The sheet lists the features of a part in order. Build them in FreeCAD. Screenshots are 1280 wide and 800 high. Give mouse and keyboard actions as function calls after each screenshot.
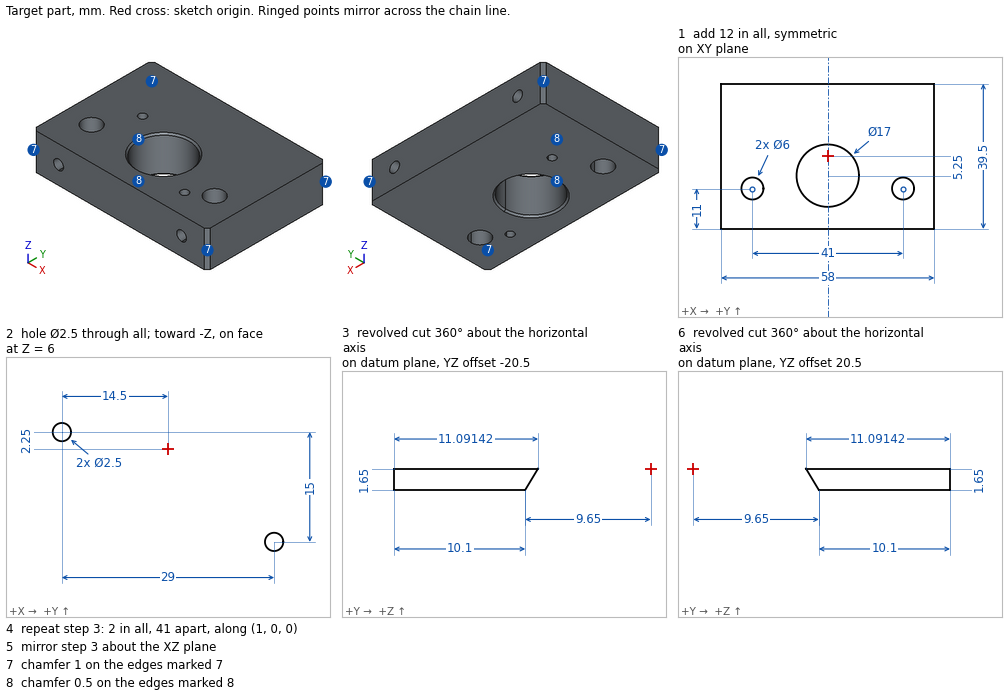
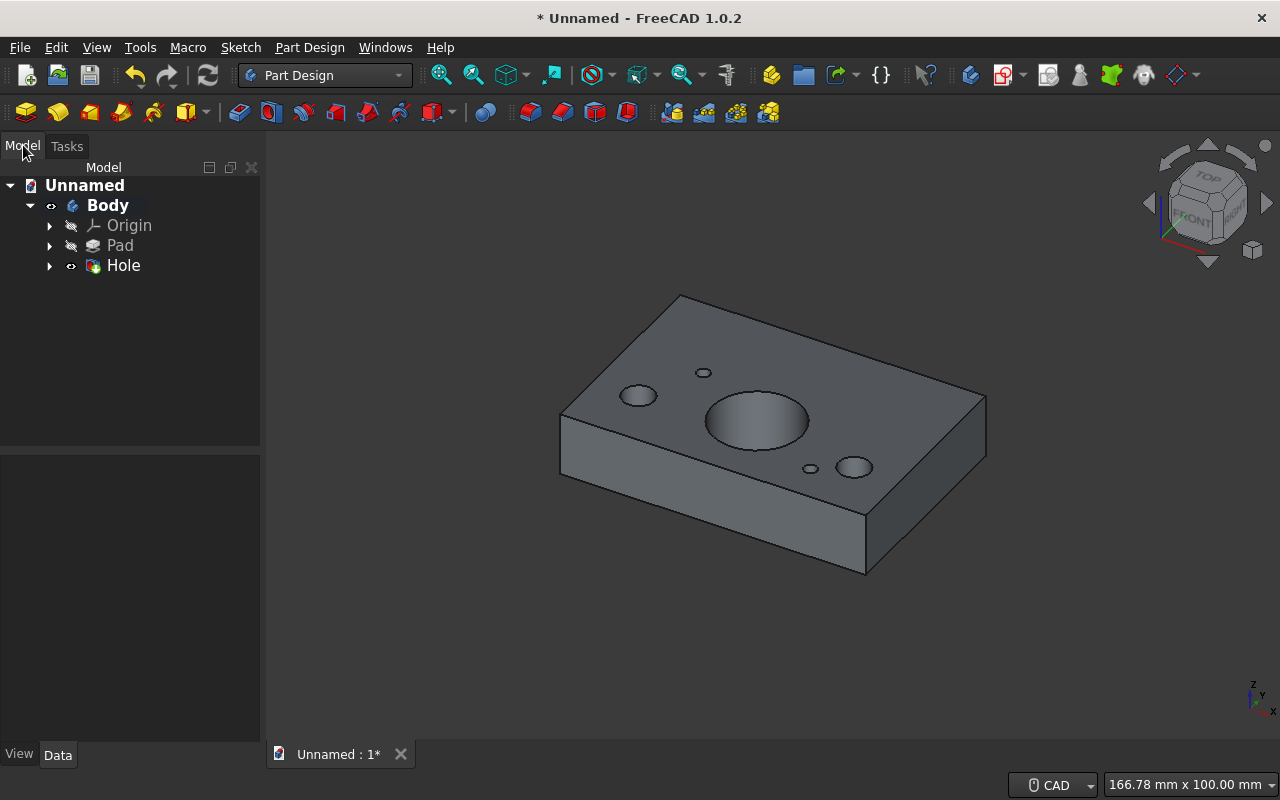
click(50, 226)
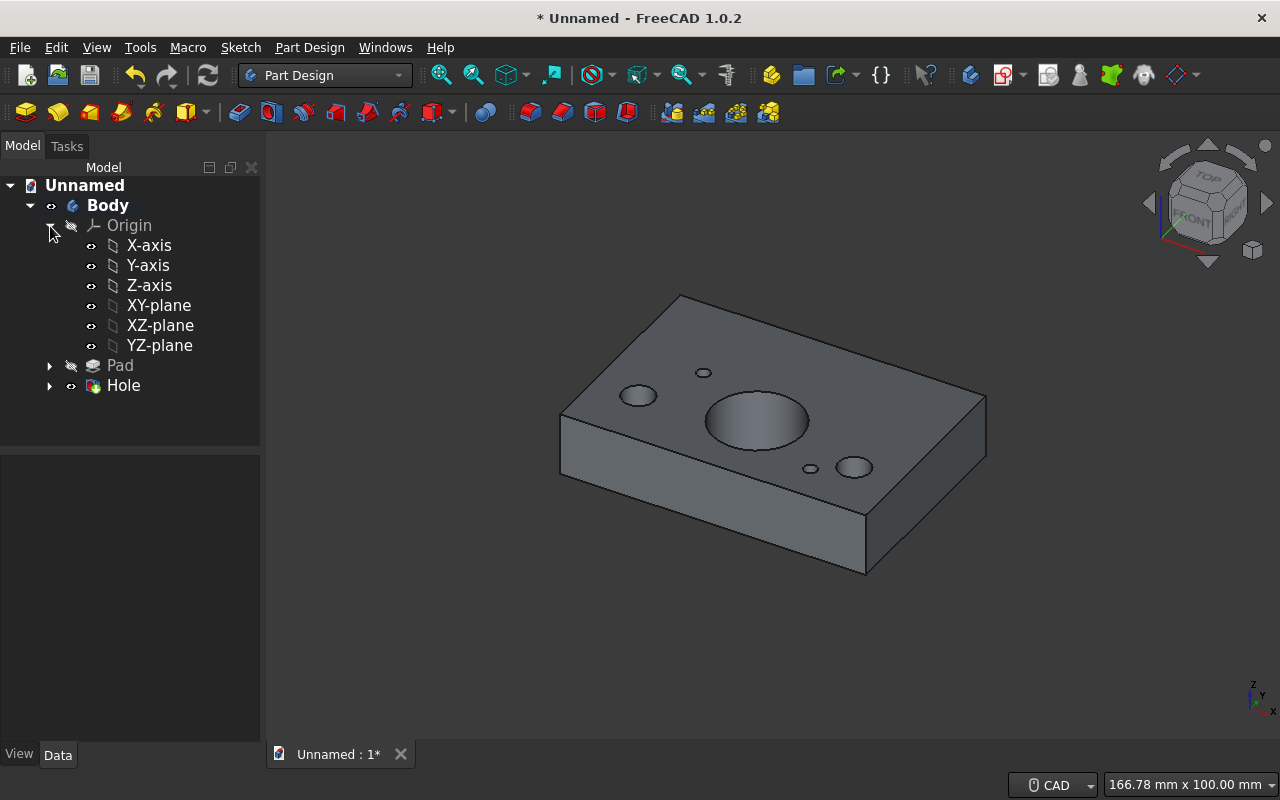
click(136, 346)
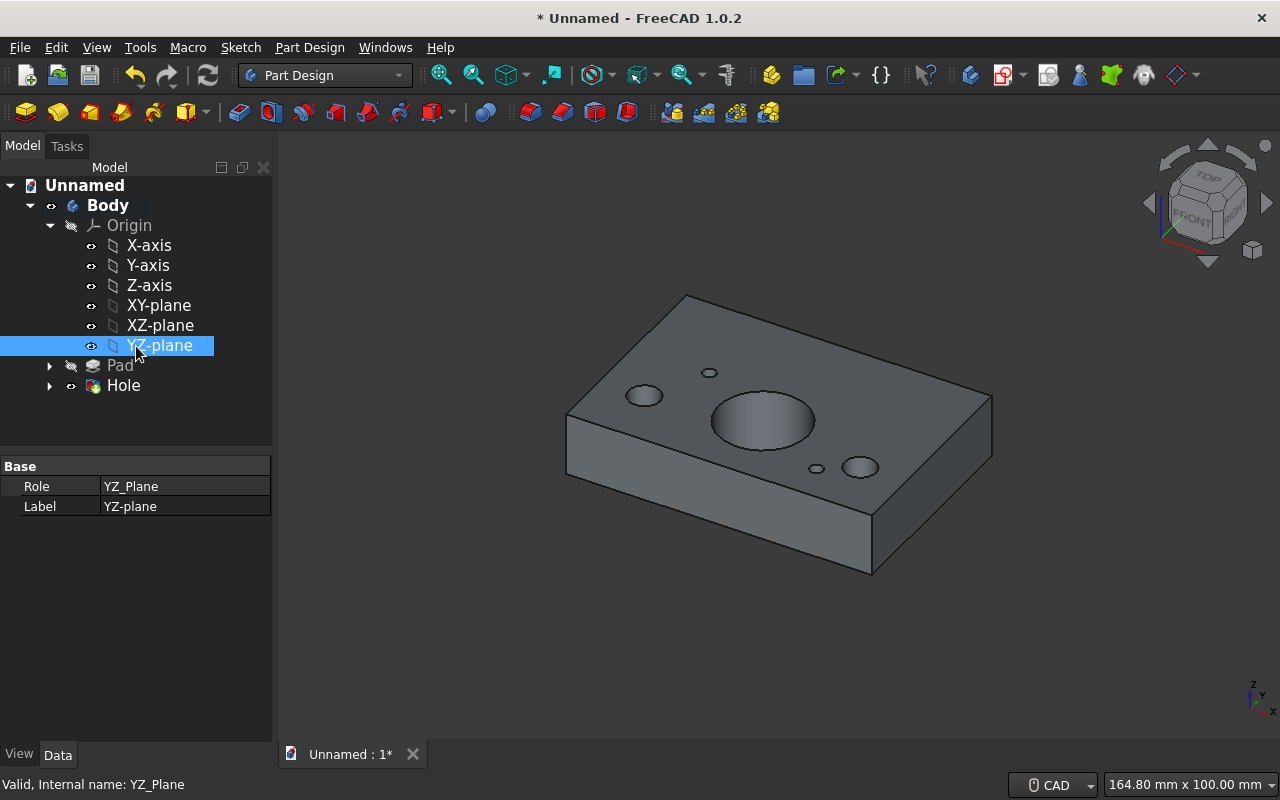
click(1176, 76)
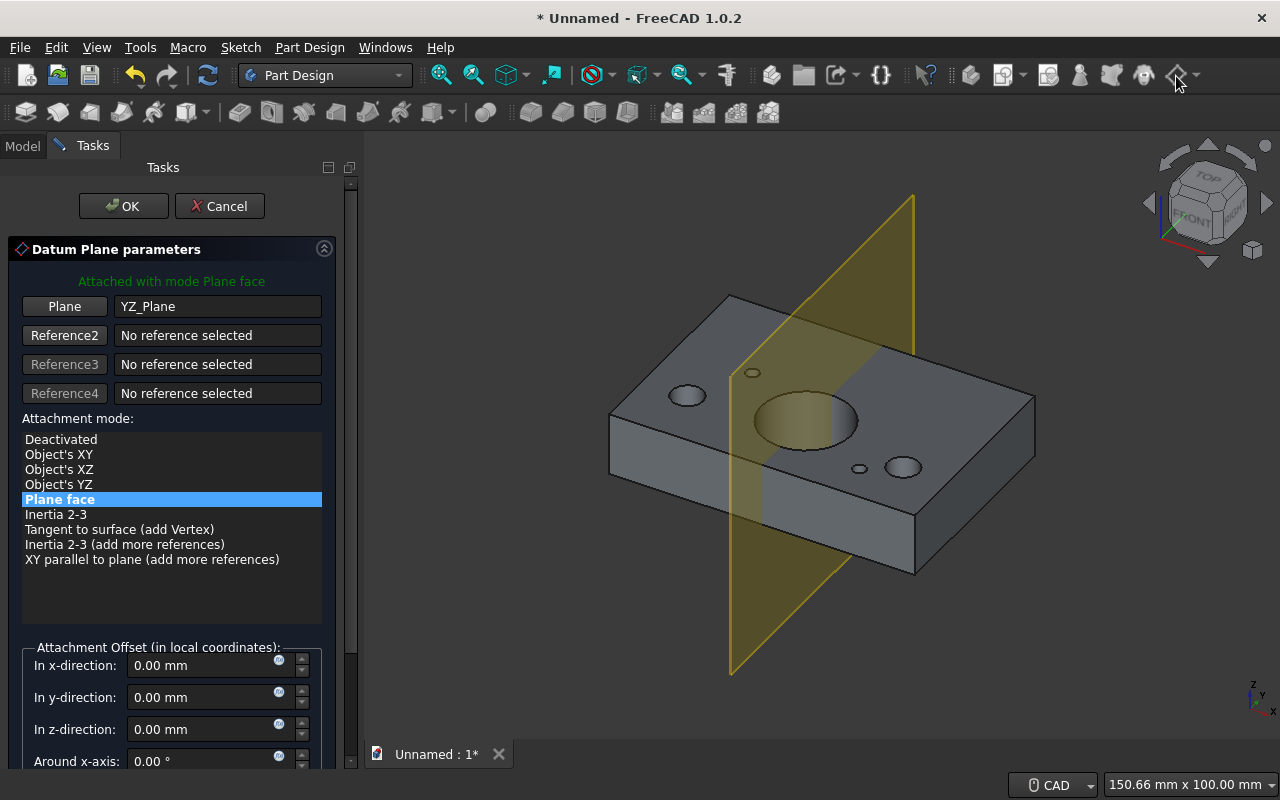
triple_click(210, 729)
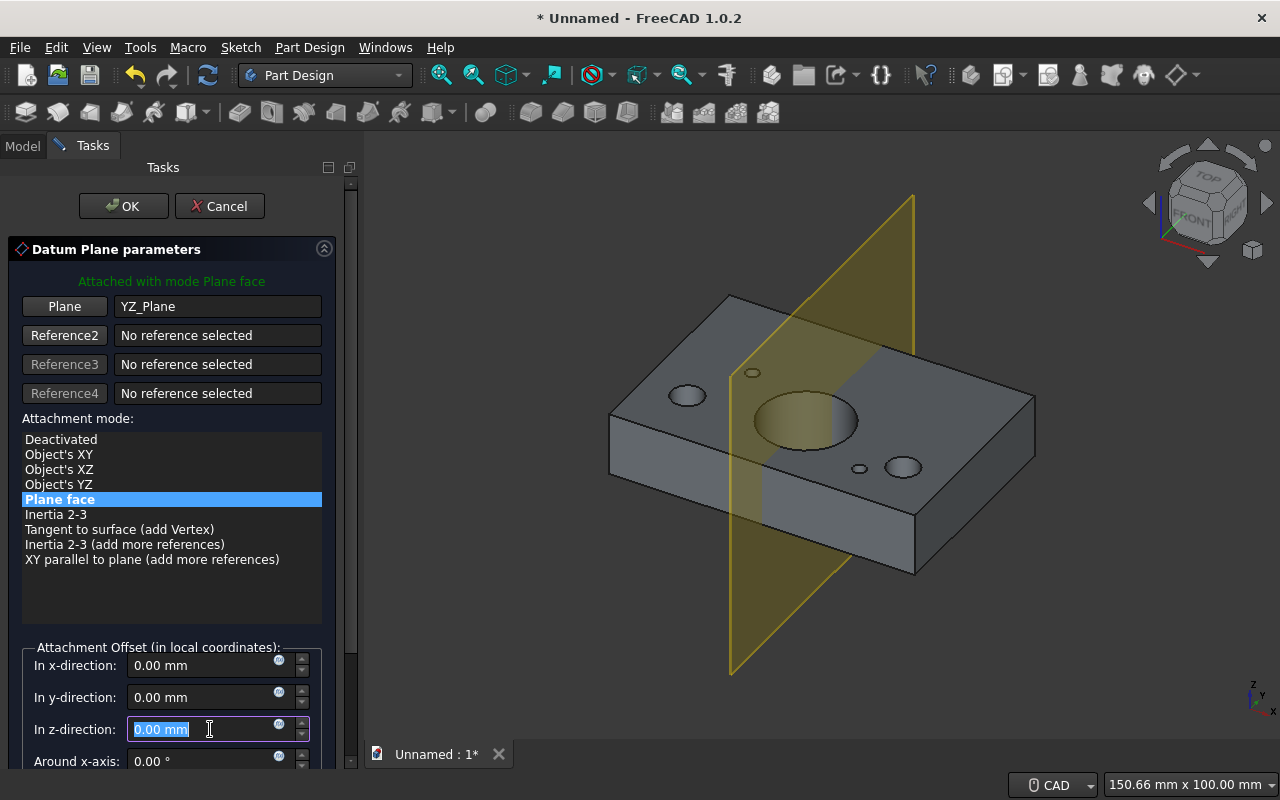
text(-20.5)
key(Tab)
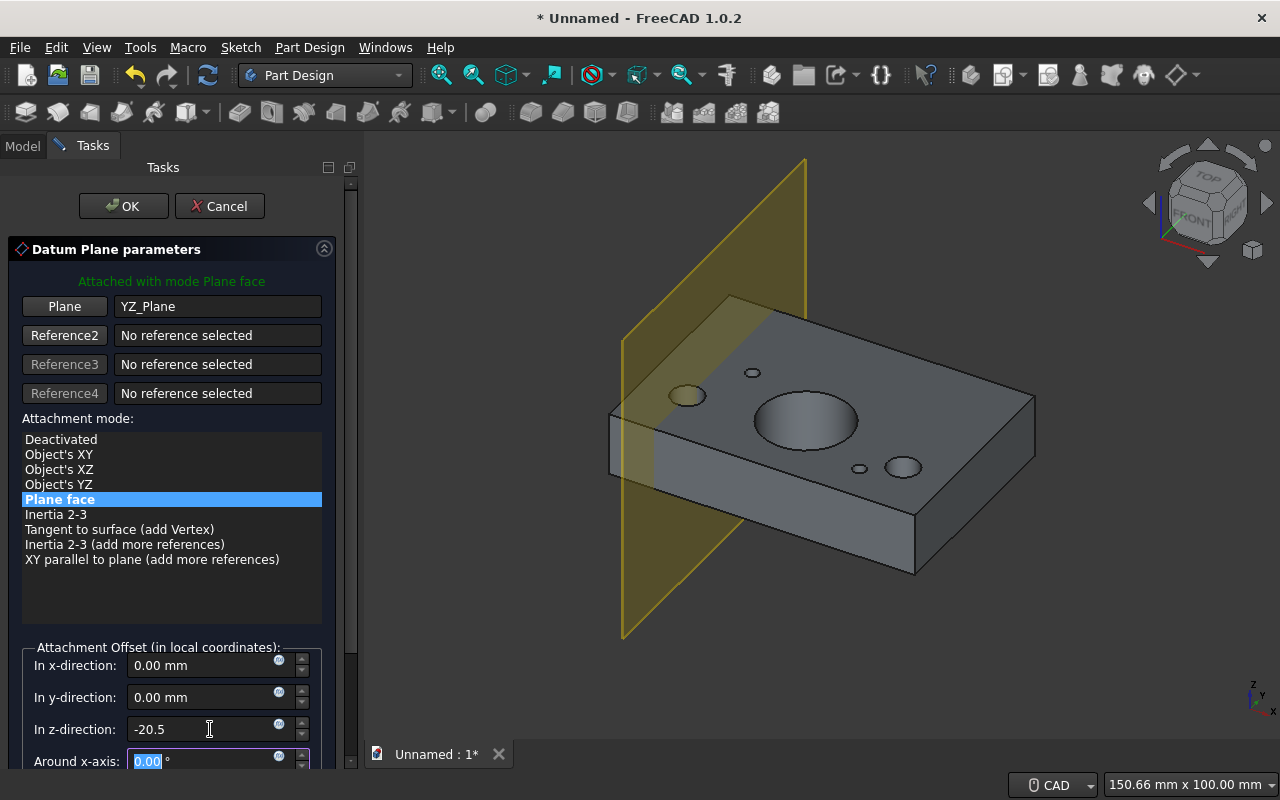
click(124, 206)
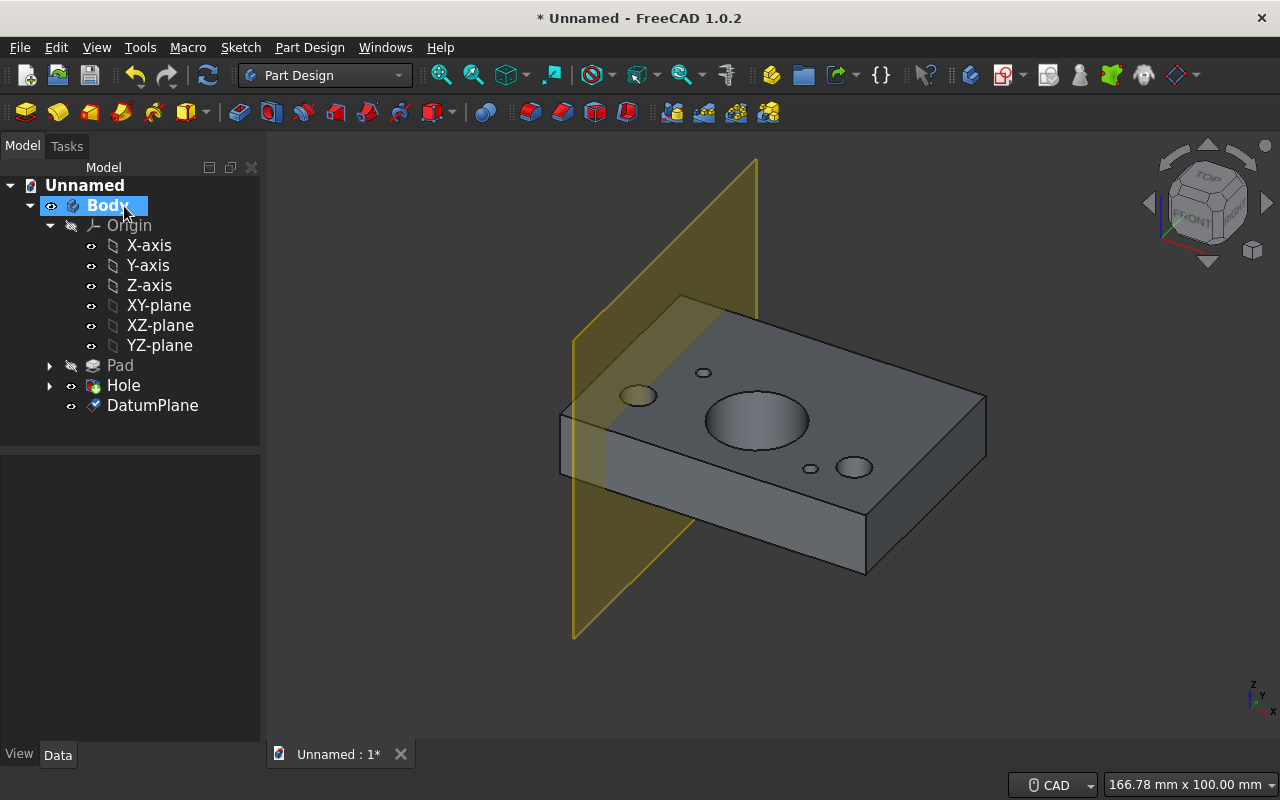
click(116, 406)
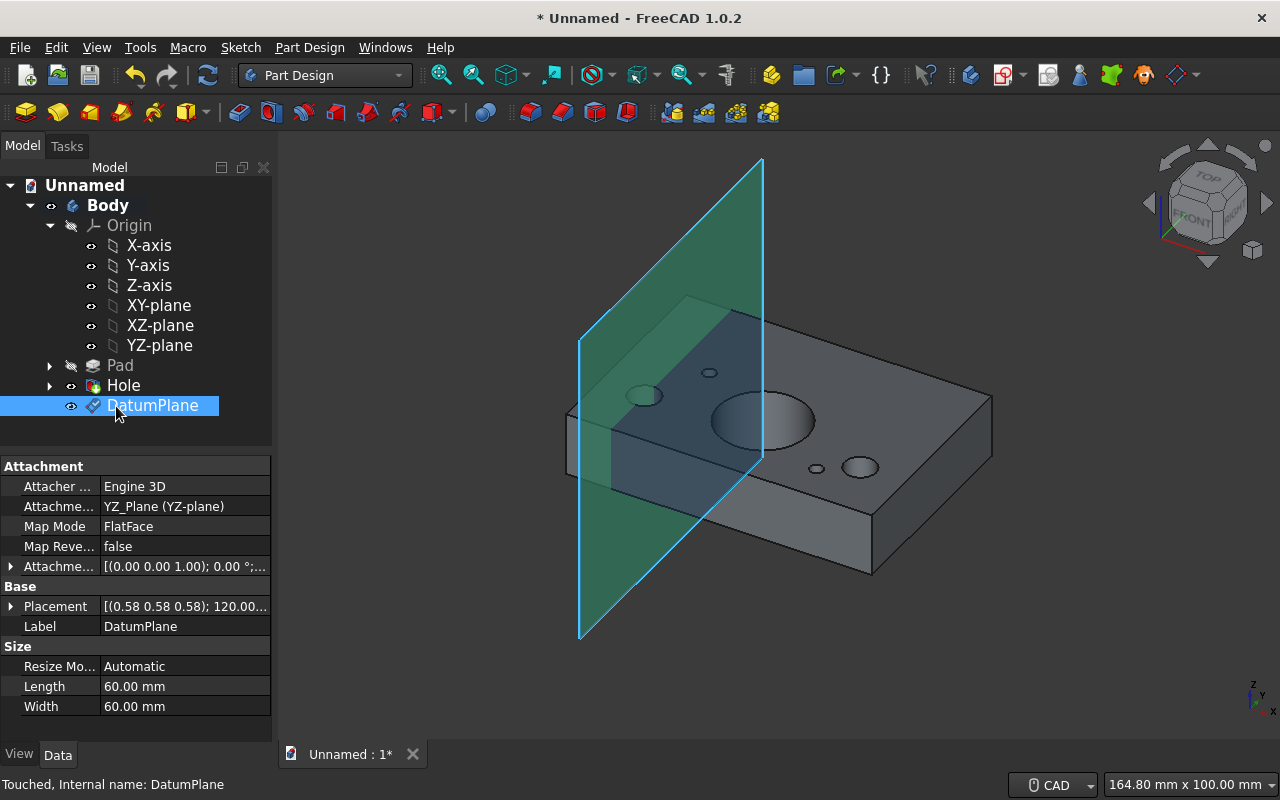
click(1004, 76)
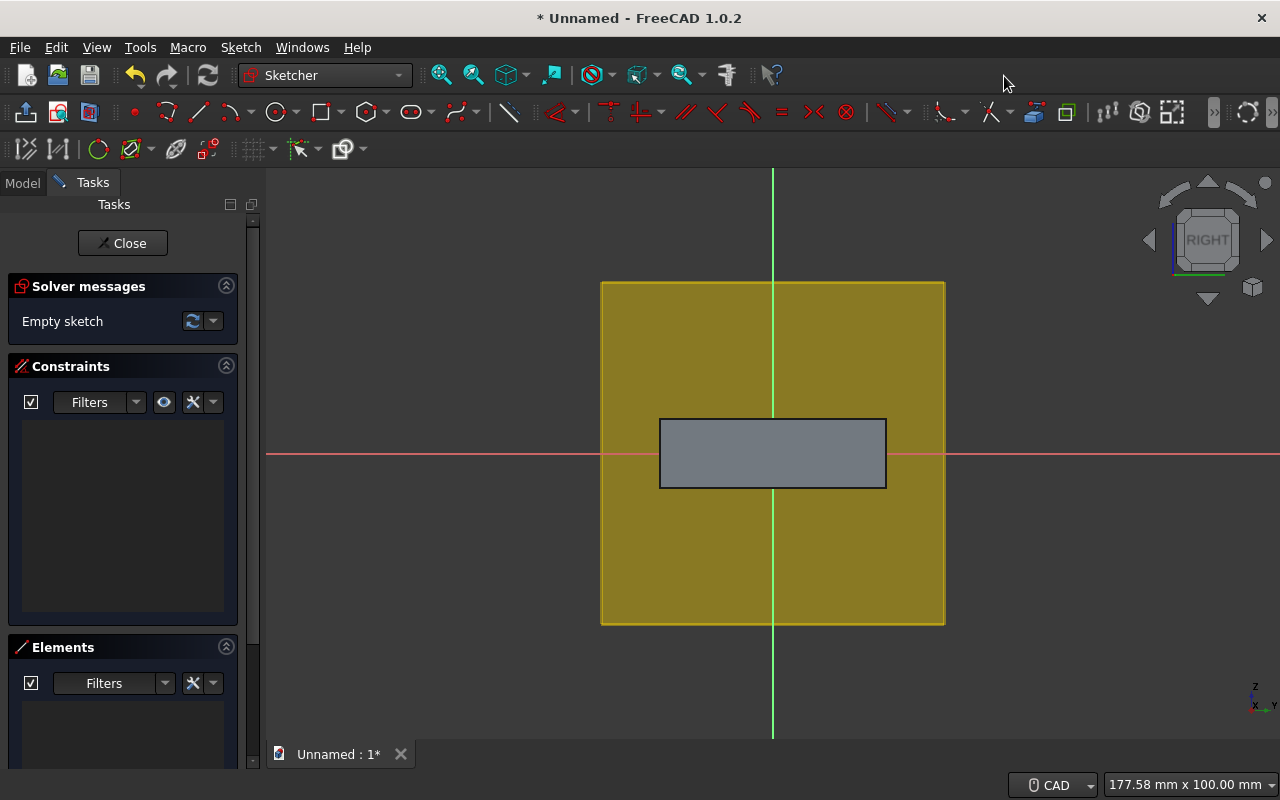
key(q)
key(s)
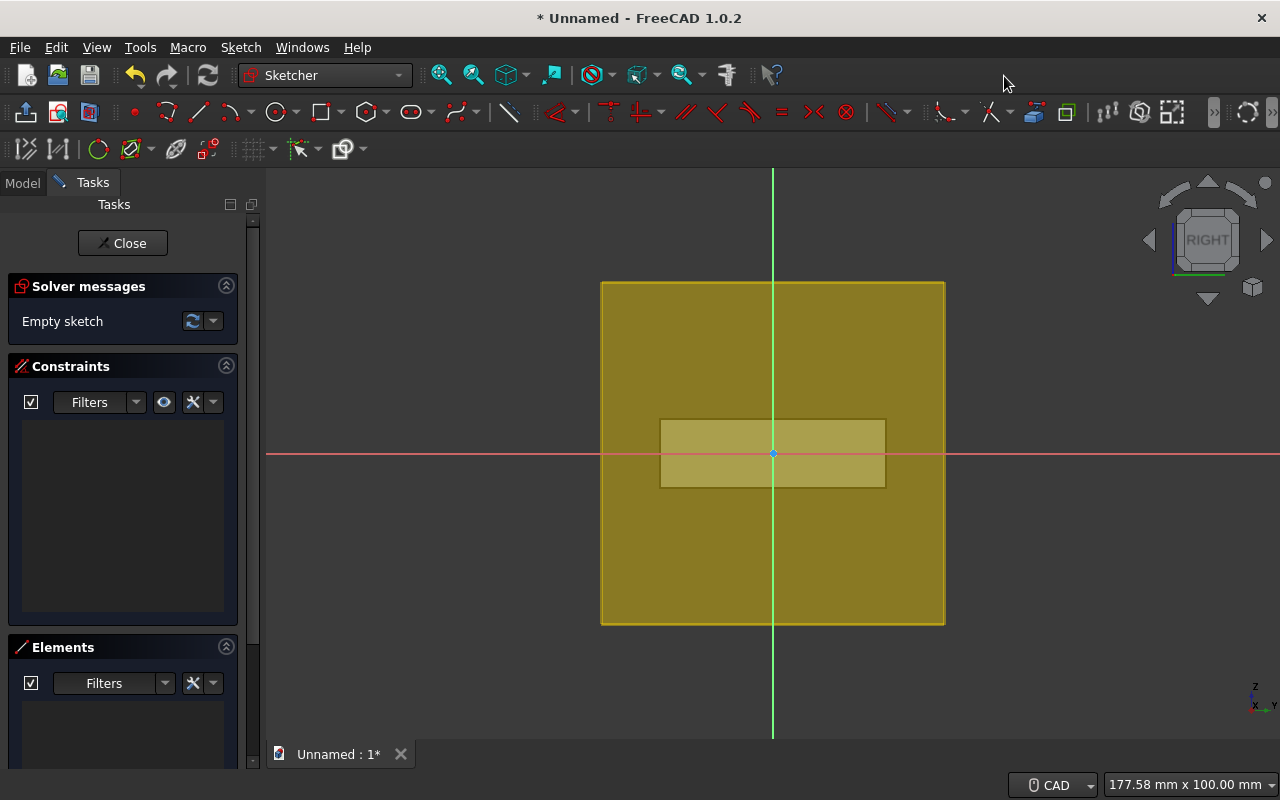
scroll(720, 459, up, 8)